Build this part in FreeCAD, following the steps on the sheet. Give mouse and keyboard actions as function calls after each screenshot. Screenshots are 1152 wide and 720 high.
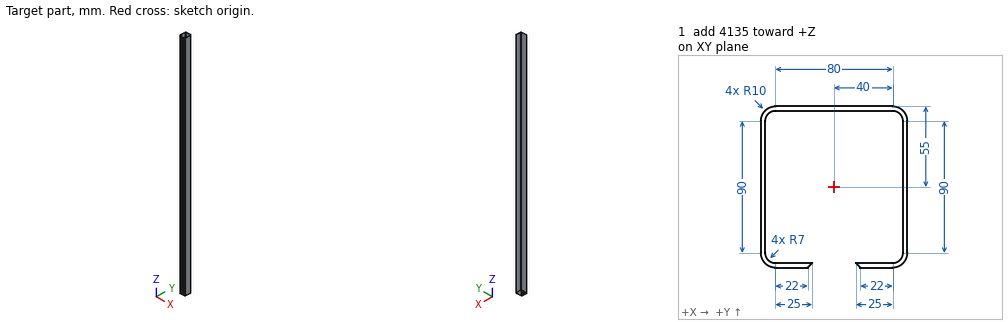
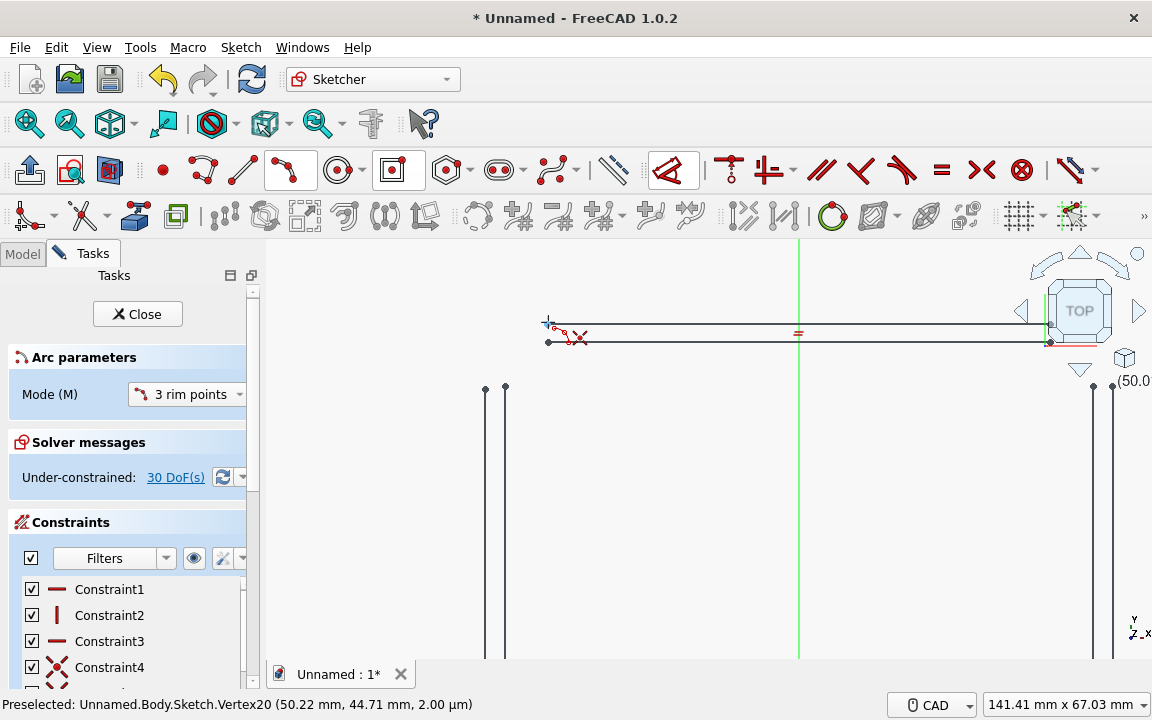
click(548, 324)
click(485, 390)
click(504, 341)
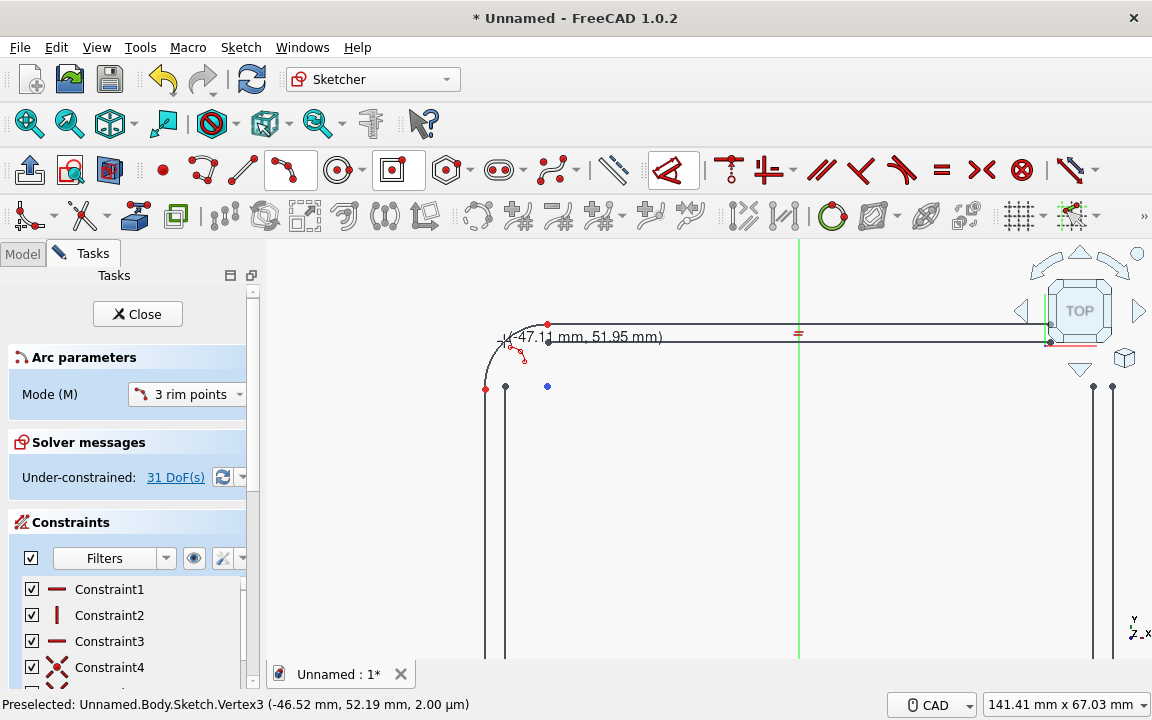
scroll(548, 322, down, 5)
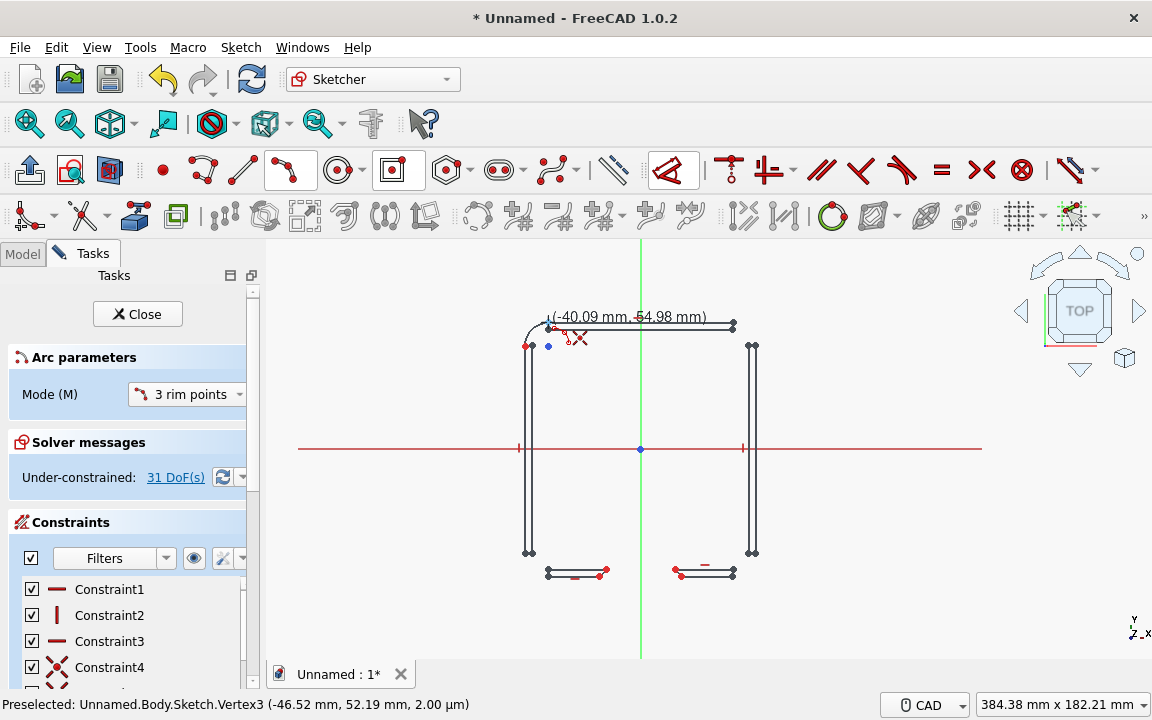
scroll(525, 553, up, 5)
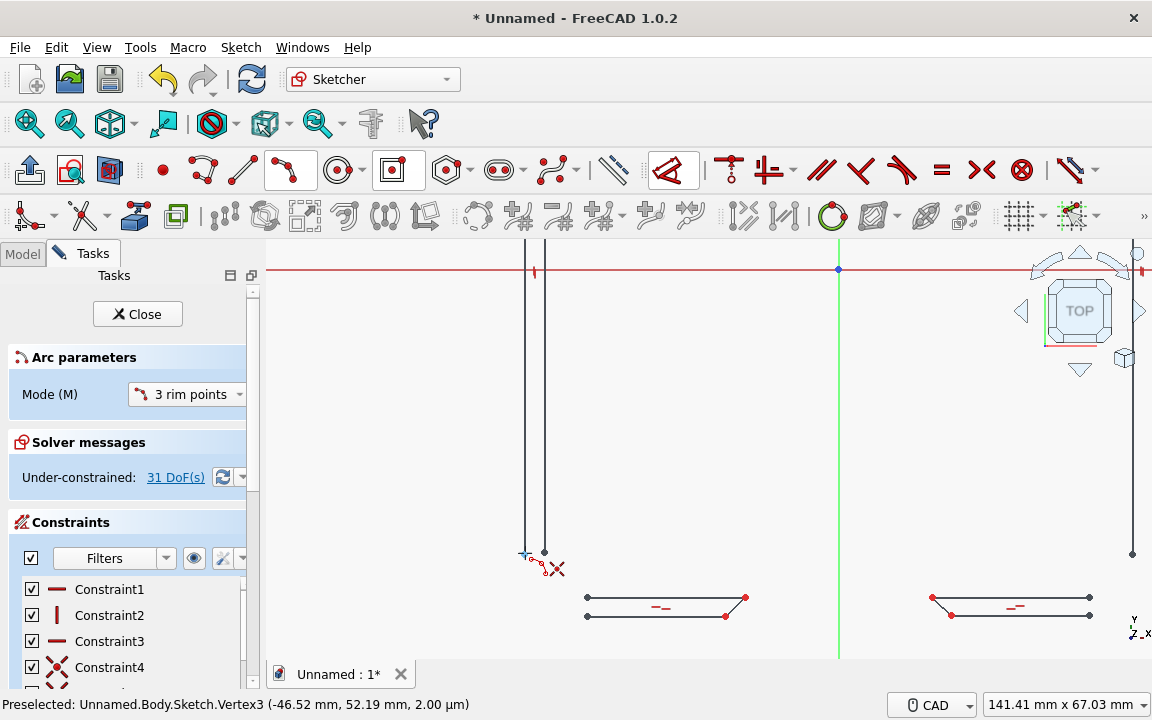
click(525, 554)
click(587, 617)
click(544, 596)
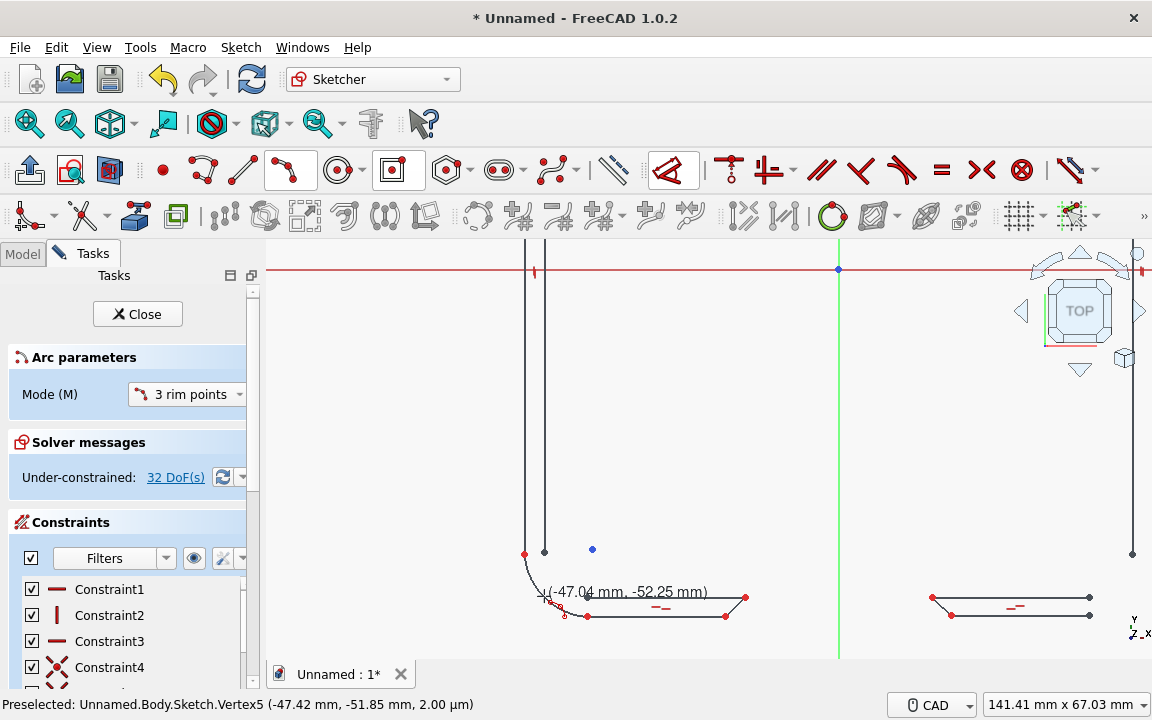
click(588, 598)
click(545, 553)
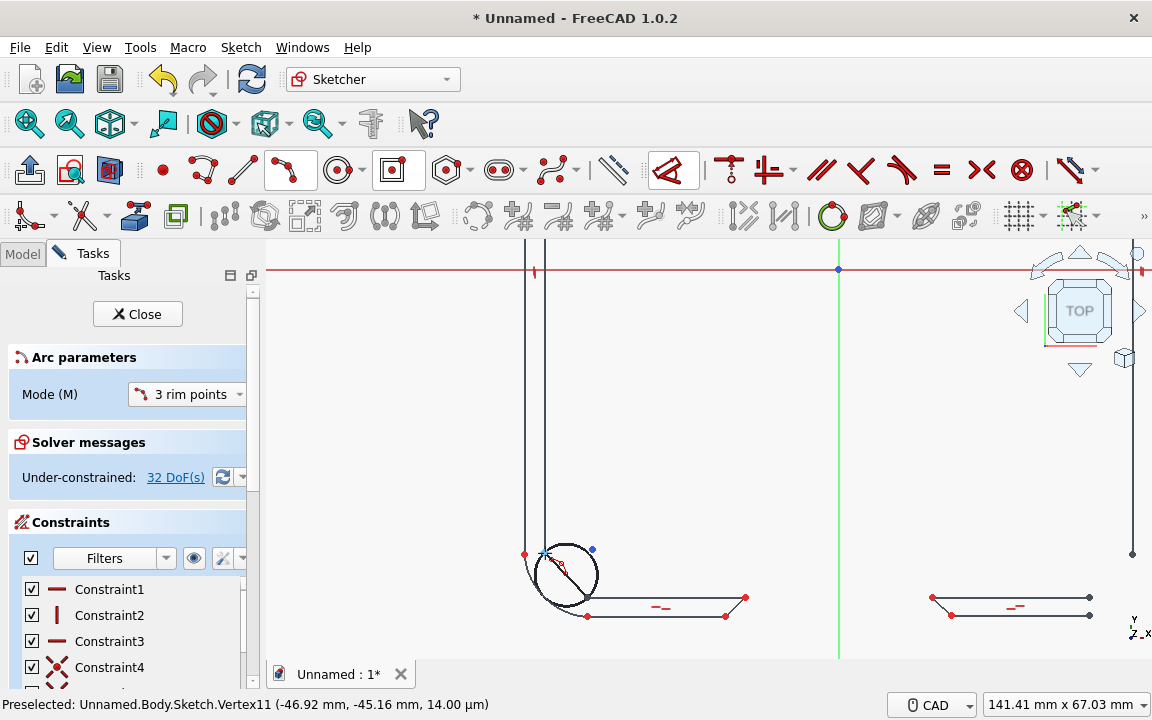
scroll(557, 583, up, 2)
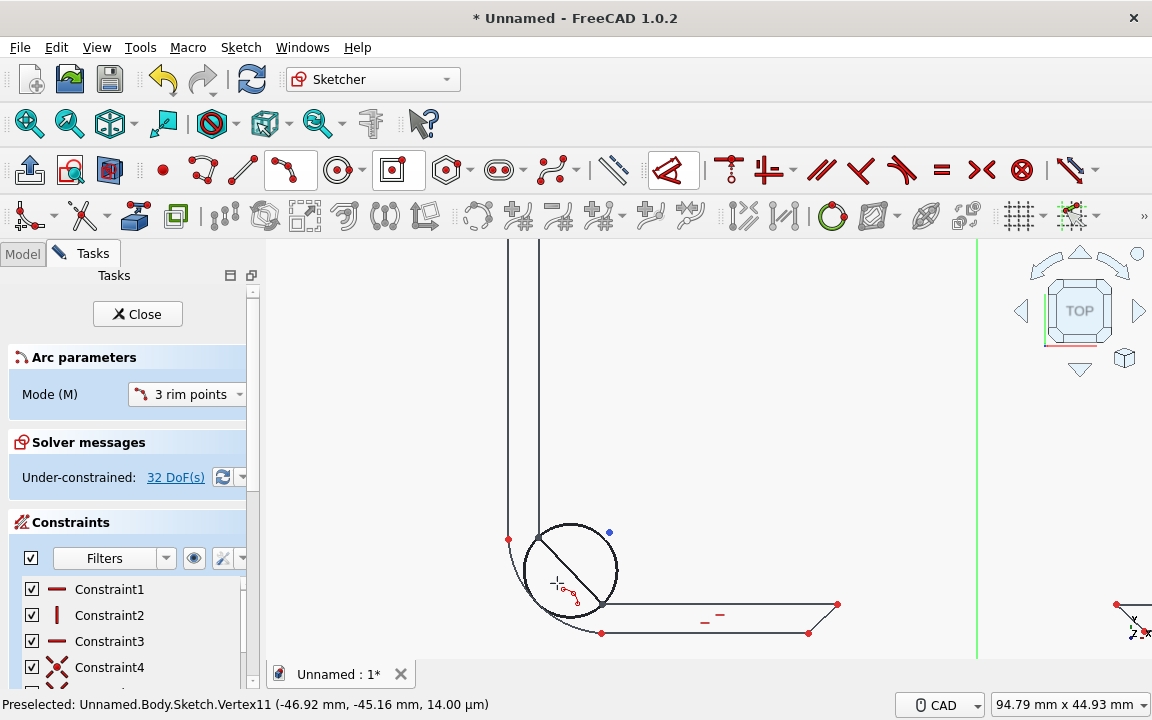
click(557, 582)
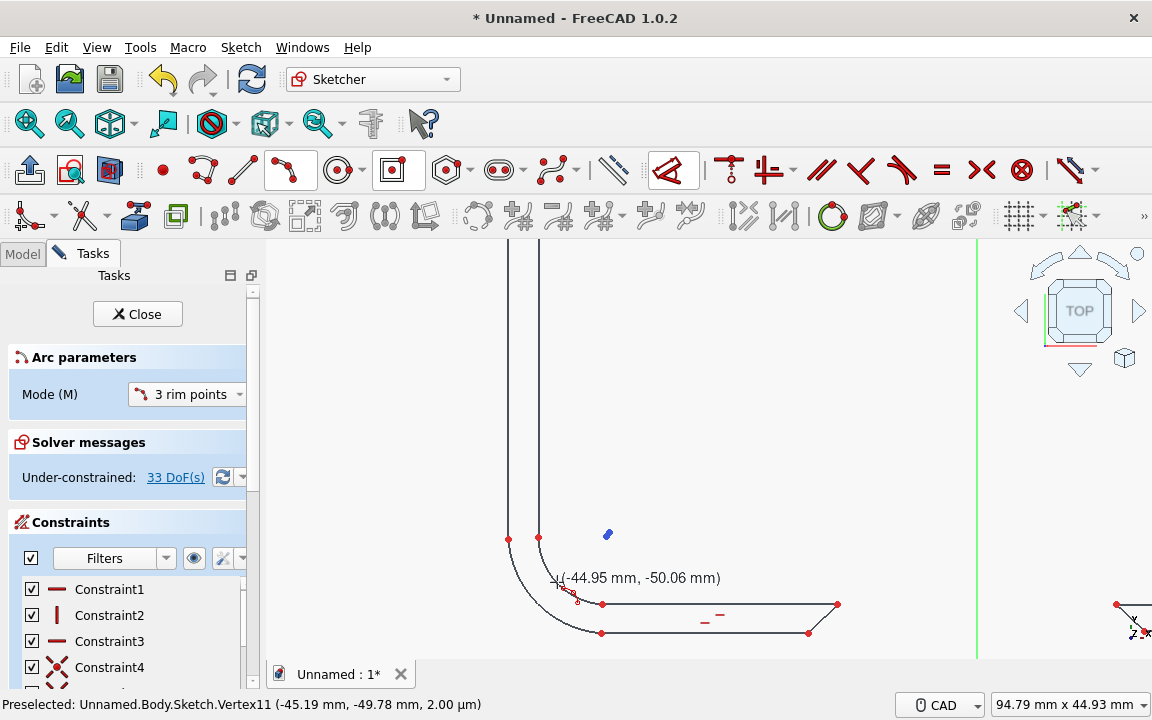
scroll(530, 558, down, 7)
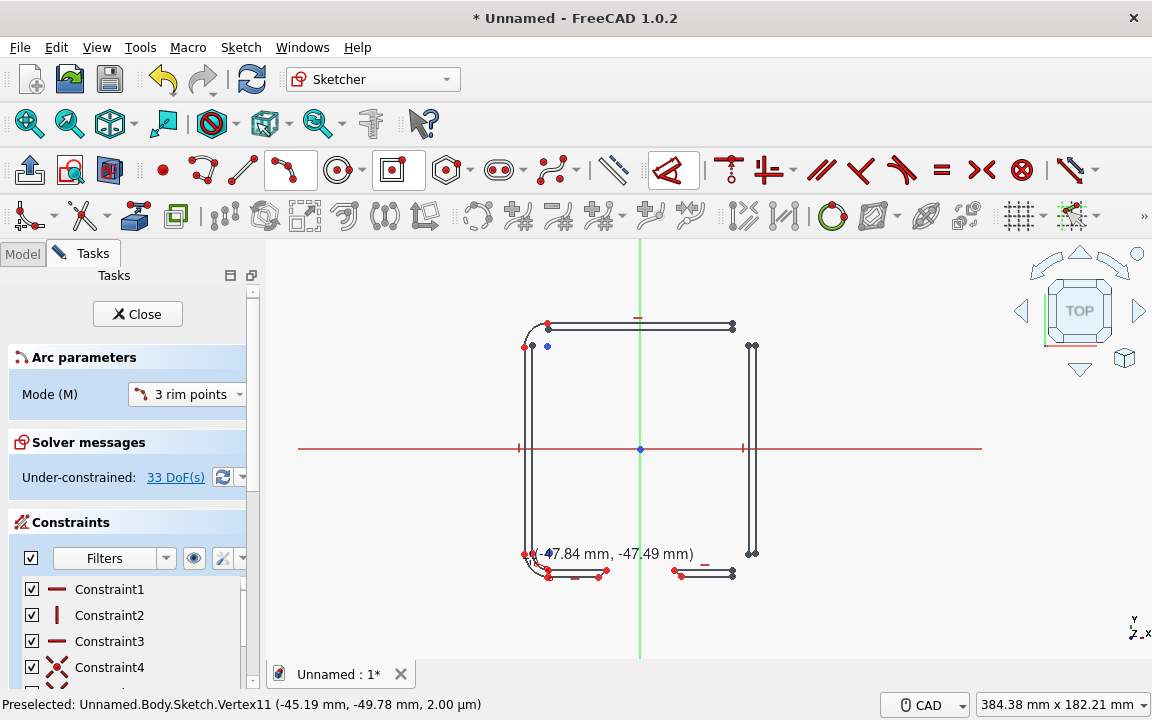
scroll(532, 346, up, 5)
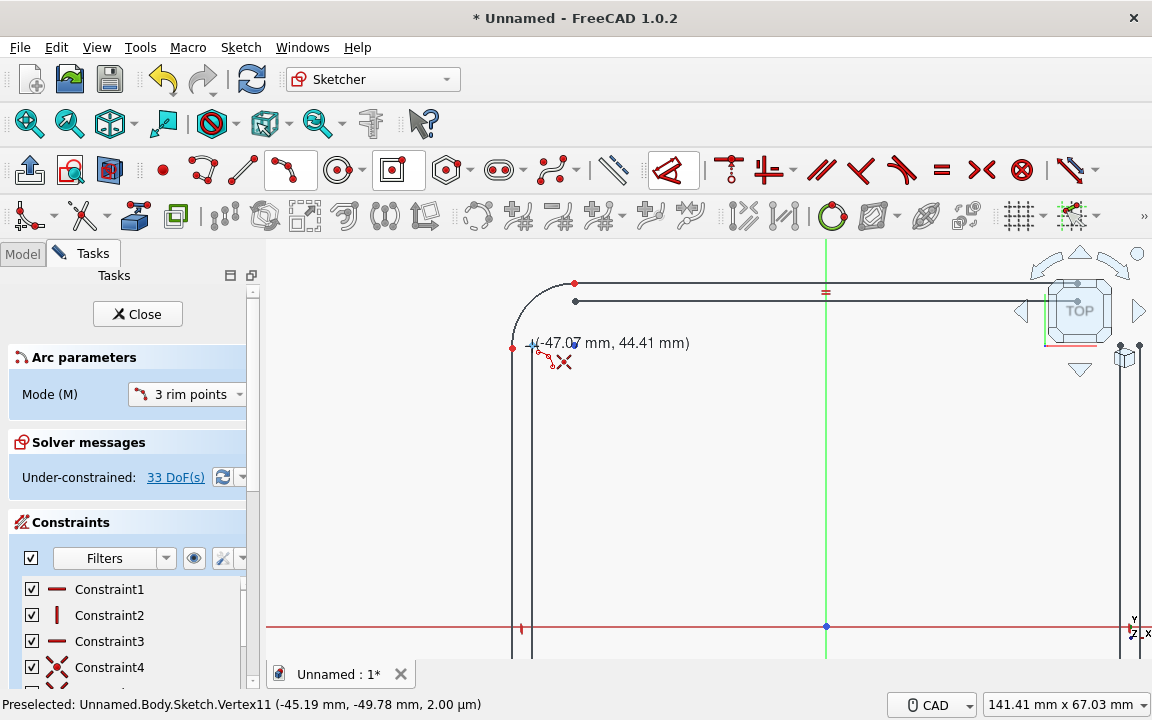
click(532, 345)
click(576, 301)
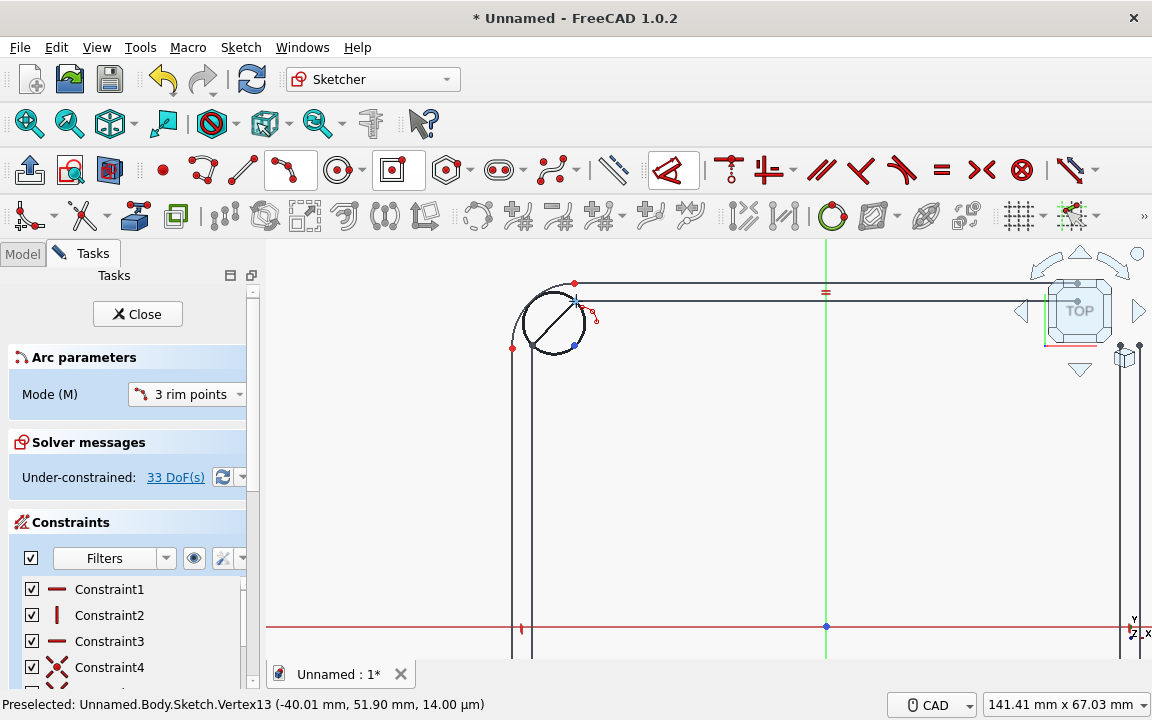
scroll(545, 314, up, 2)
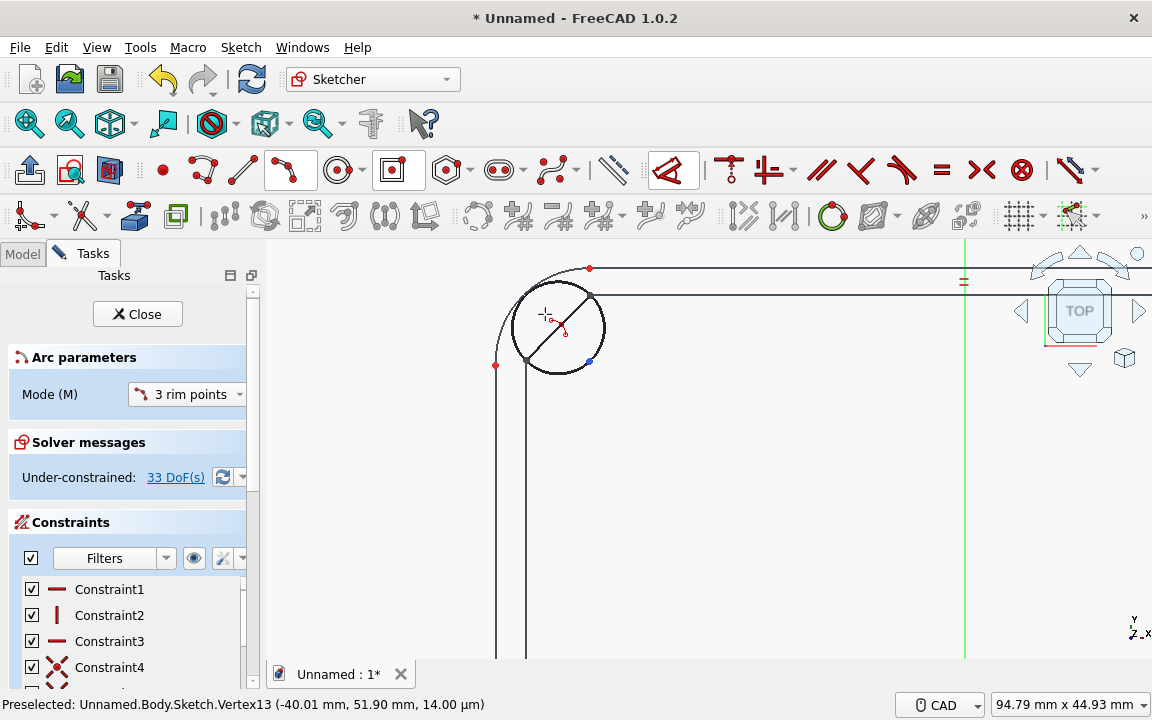
click(544, 313)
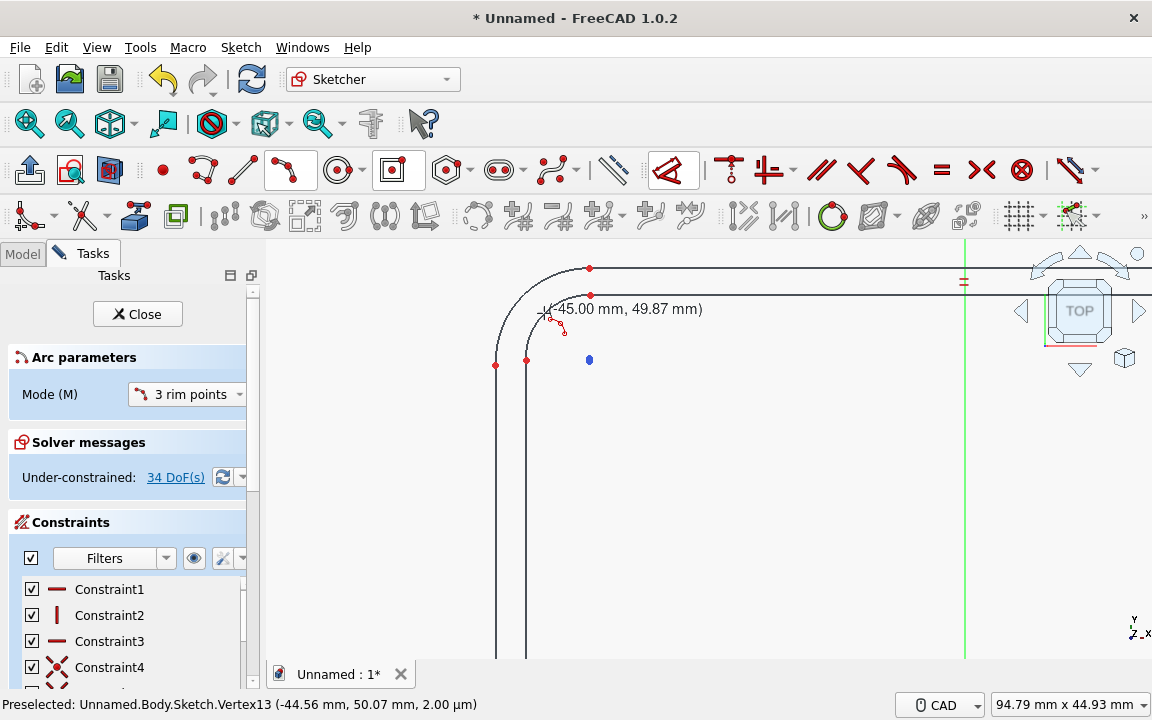
scroll(534, 341, down, 7)